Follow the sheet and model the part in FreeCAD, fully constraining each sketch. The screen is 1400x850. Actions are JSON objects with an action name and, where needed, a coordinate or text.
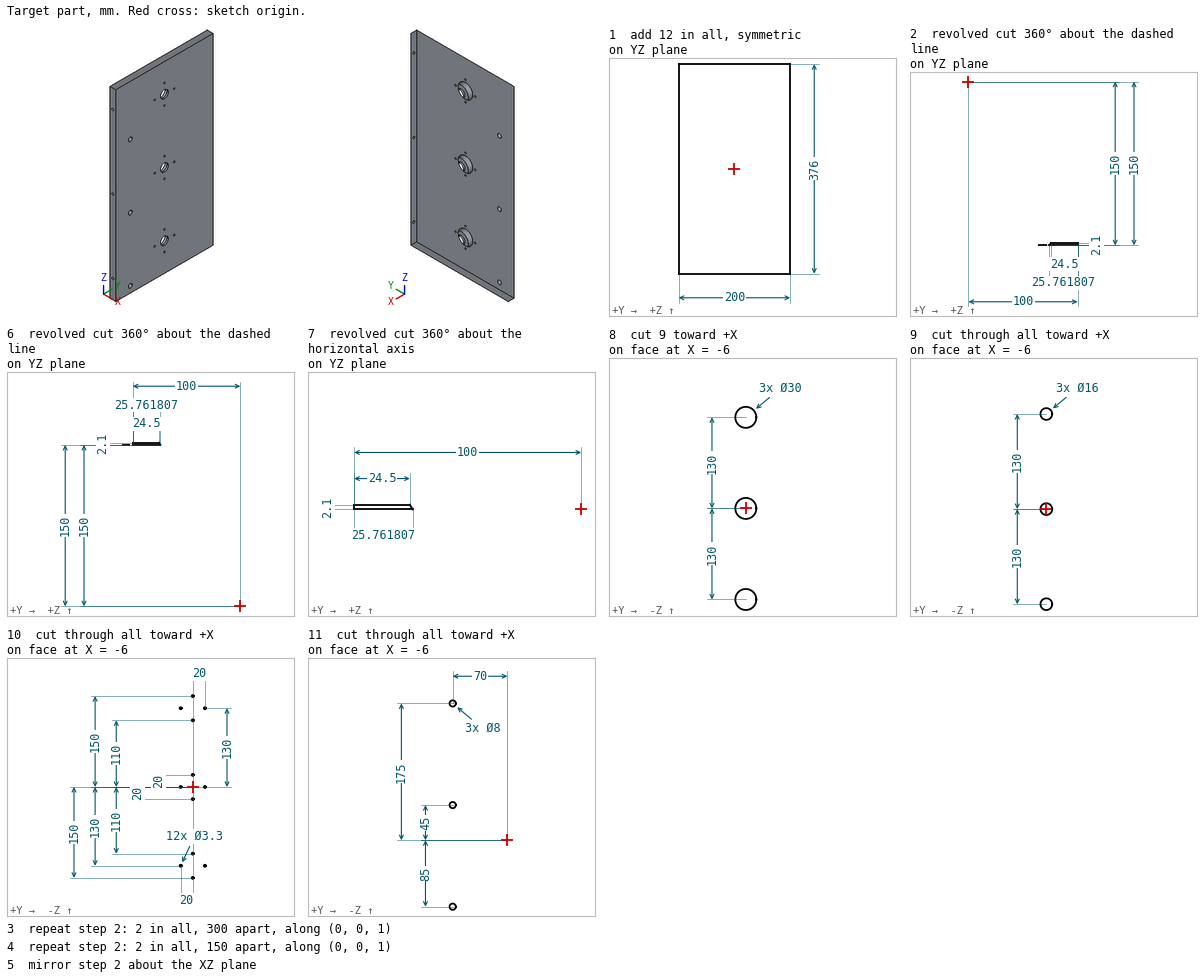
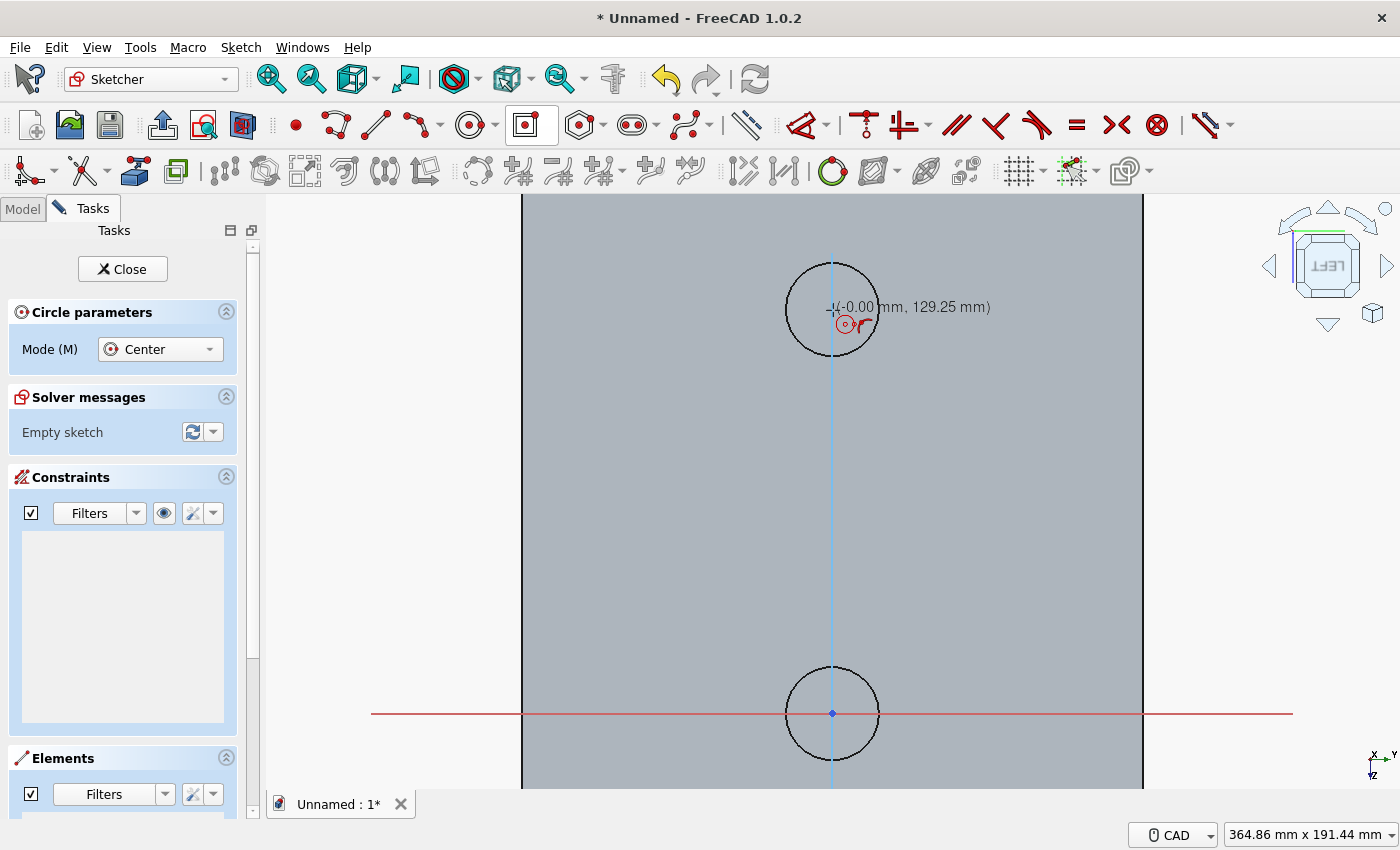
{"action": "left_click", "coordinate": [832, 310]}
{"action": "mouse_move", "coordinate": [850, 292]}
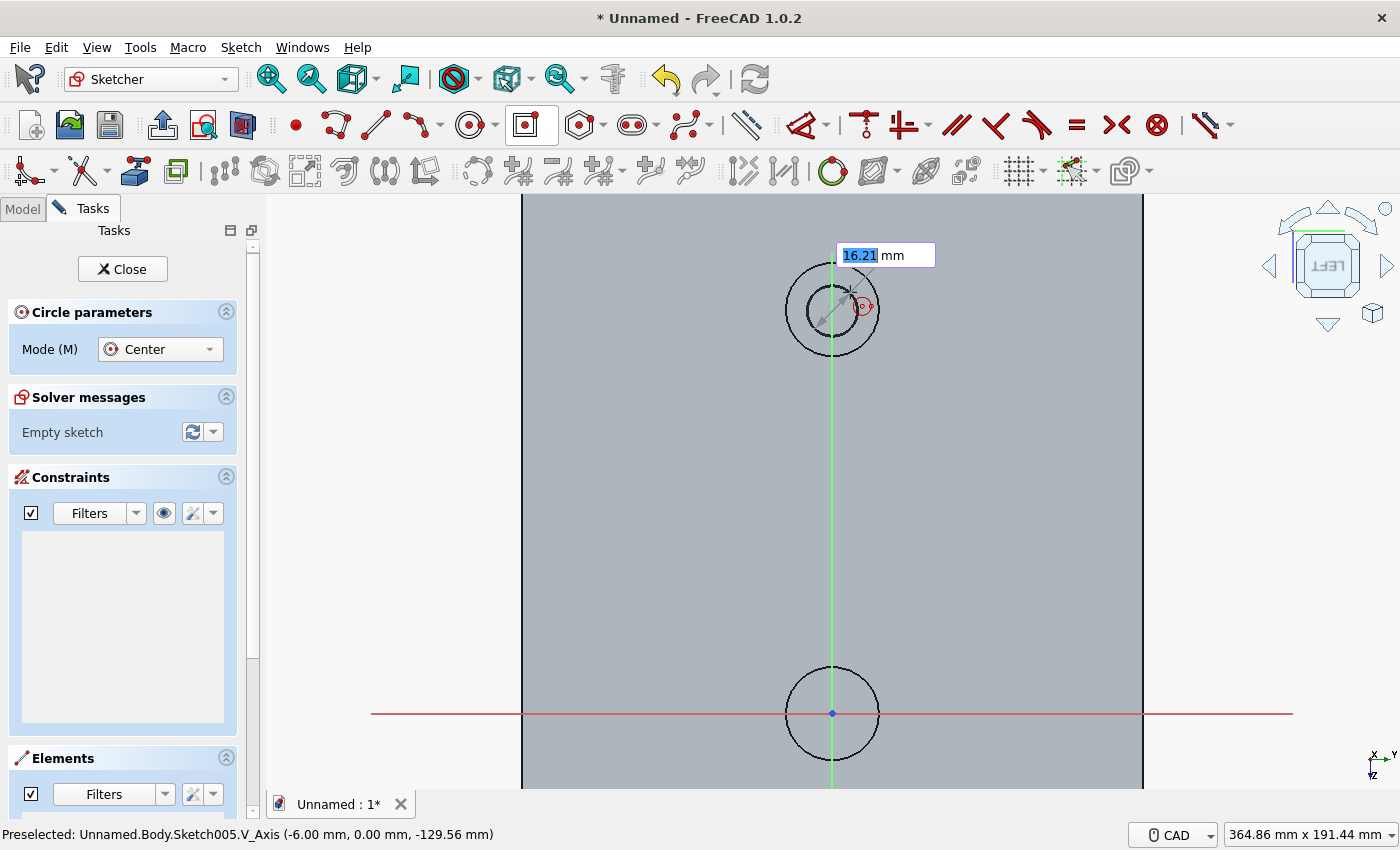
{"action": "type", "text": "16"}
{"action": "key", "text": "Return"}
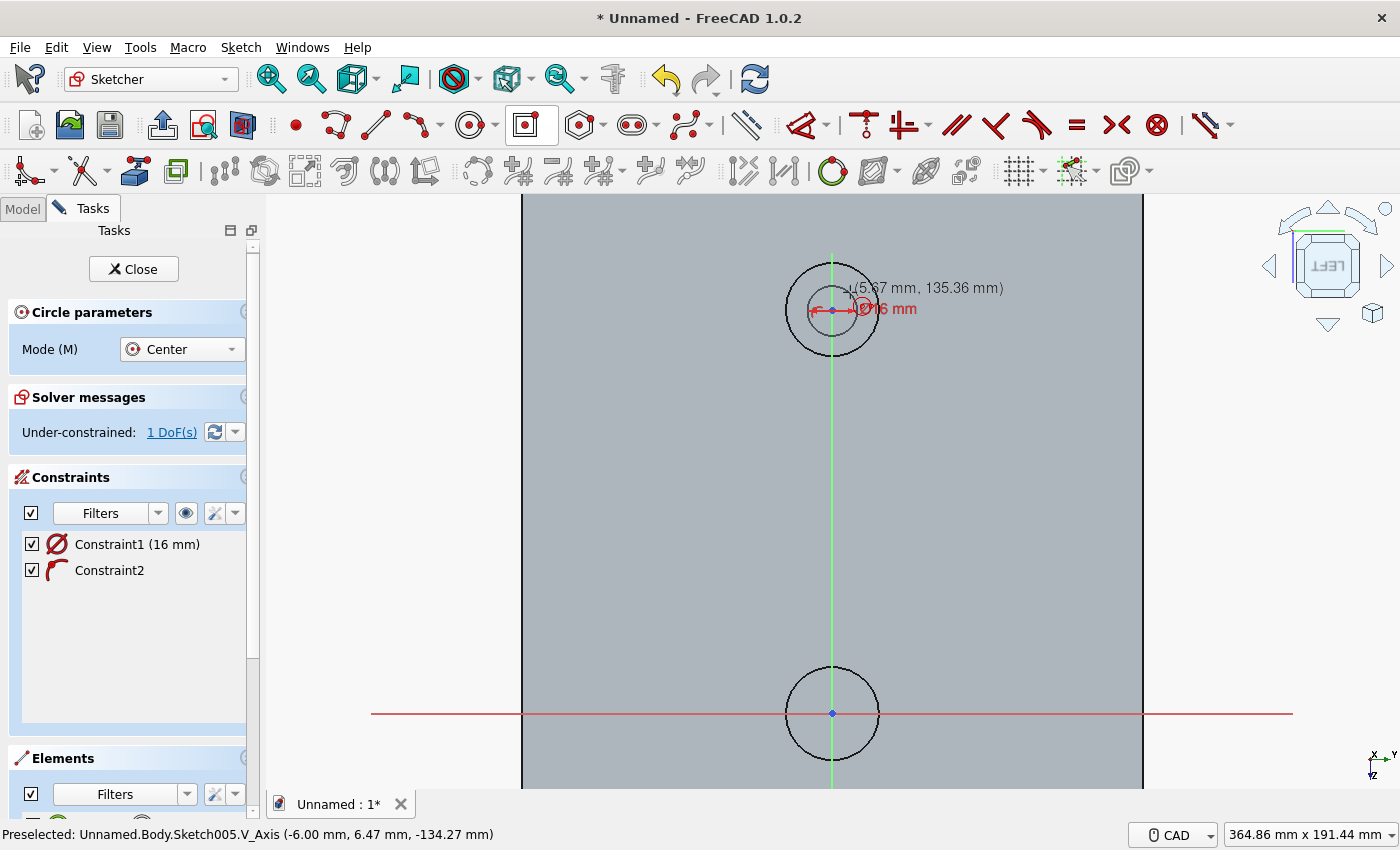
{"action": "left_click", "coordinate": [832, 714]}
{"action": "mouse_move", "coordinate": [850, 696]}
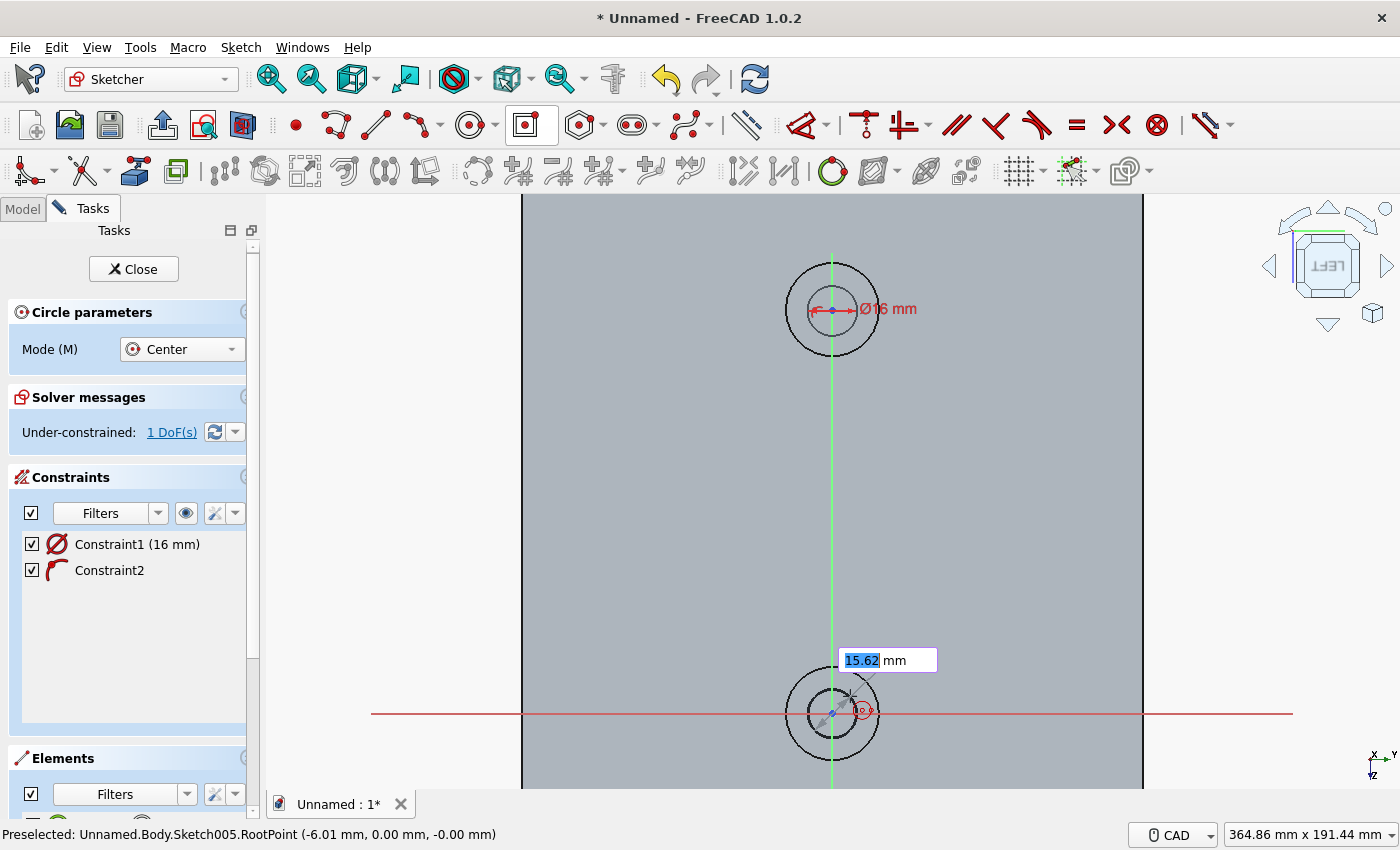
{"action": "type", "text": "16"}
{"action": "key", "text": "Return"}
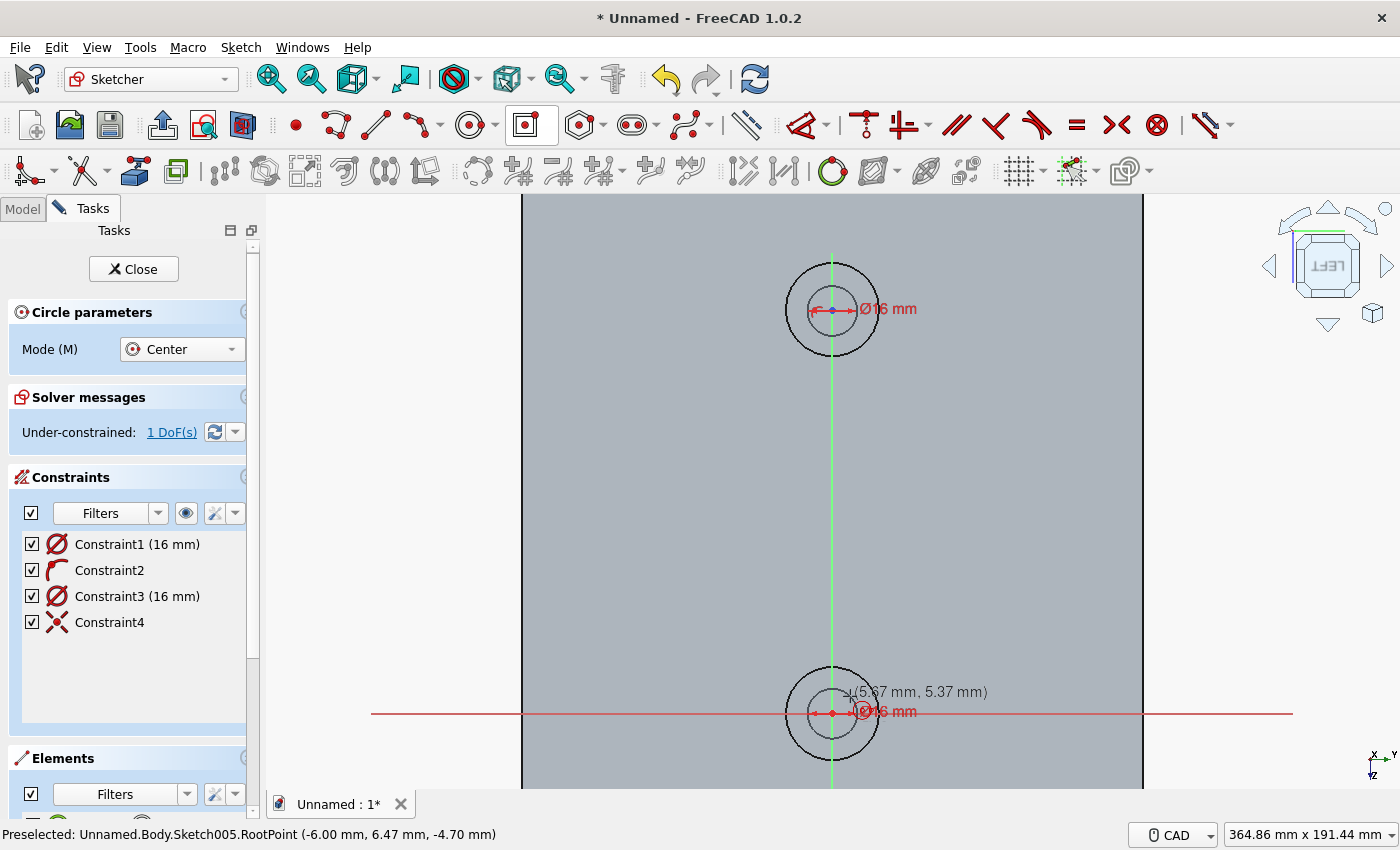
{"action": "scroll", "coordinate": [709, 310], "scroll_direction": "down", "scroll_amount": 4}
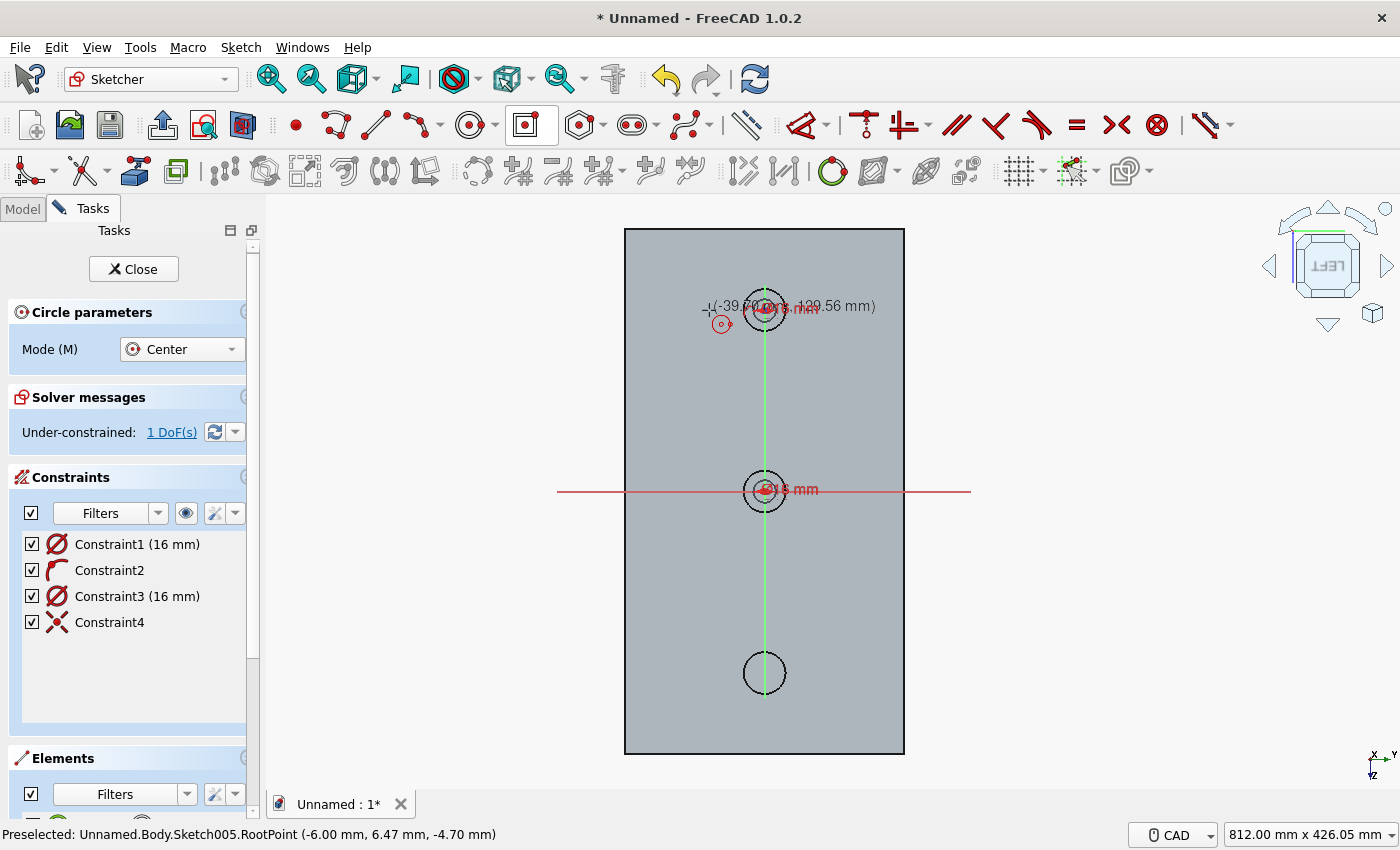
{"action": "scroll", "coordinate": [765, 673], "scroll_direction": "up", "scroll_amount": 4}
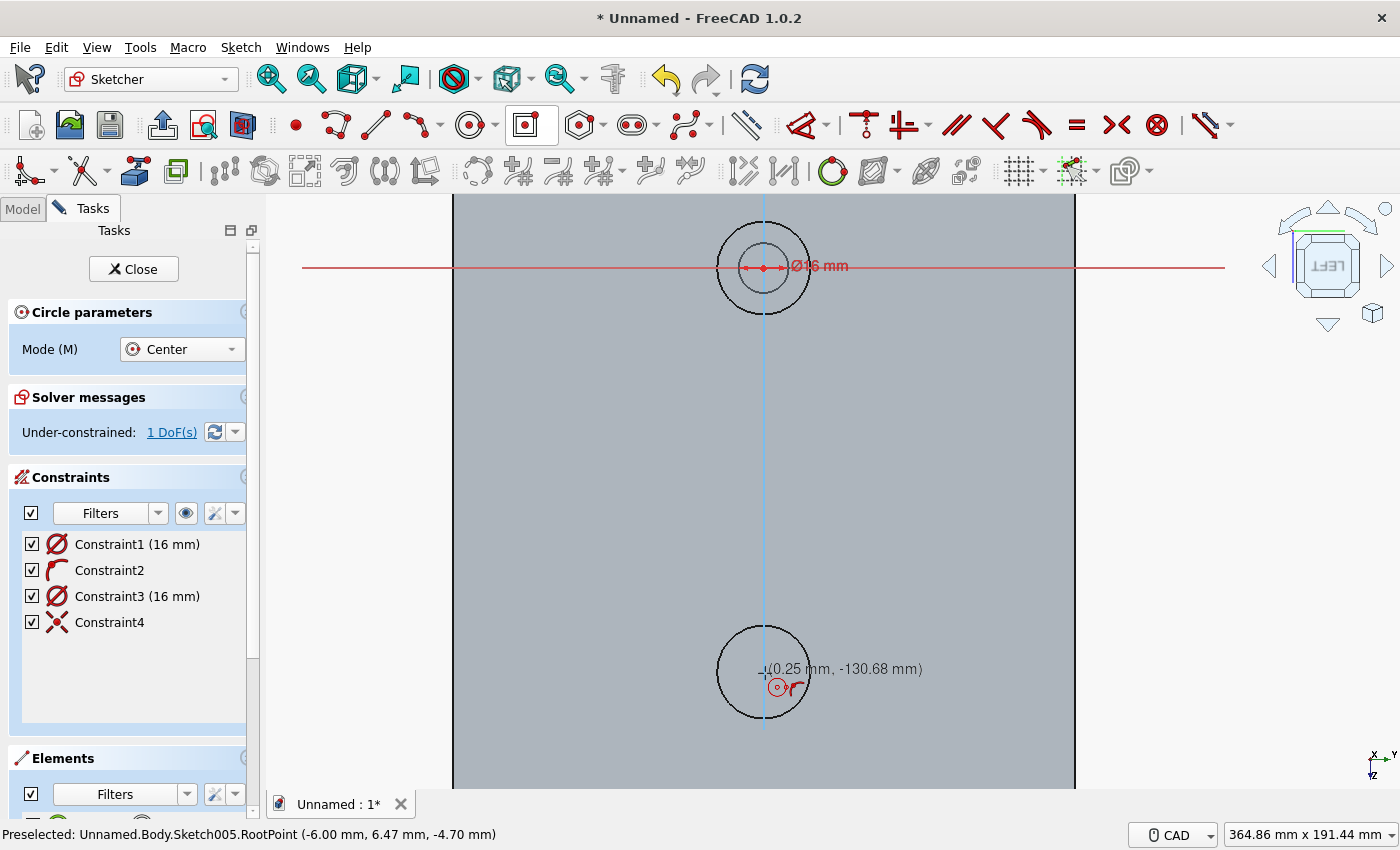
{"action": "left_click", "coordinate": [764, 672]}
{"action": "mouse_move", "coordinate": [781, 655]}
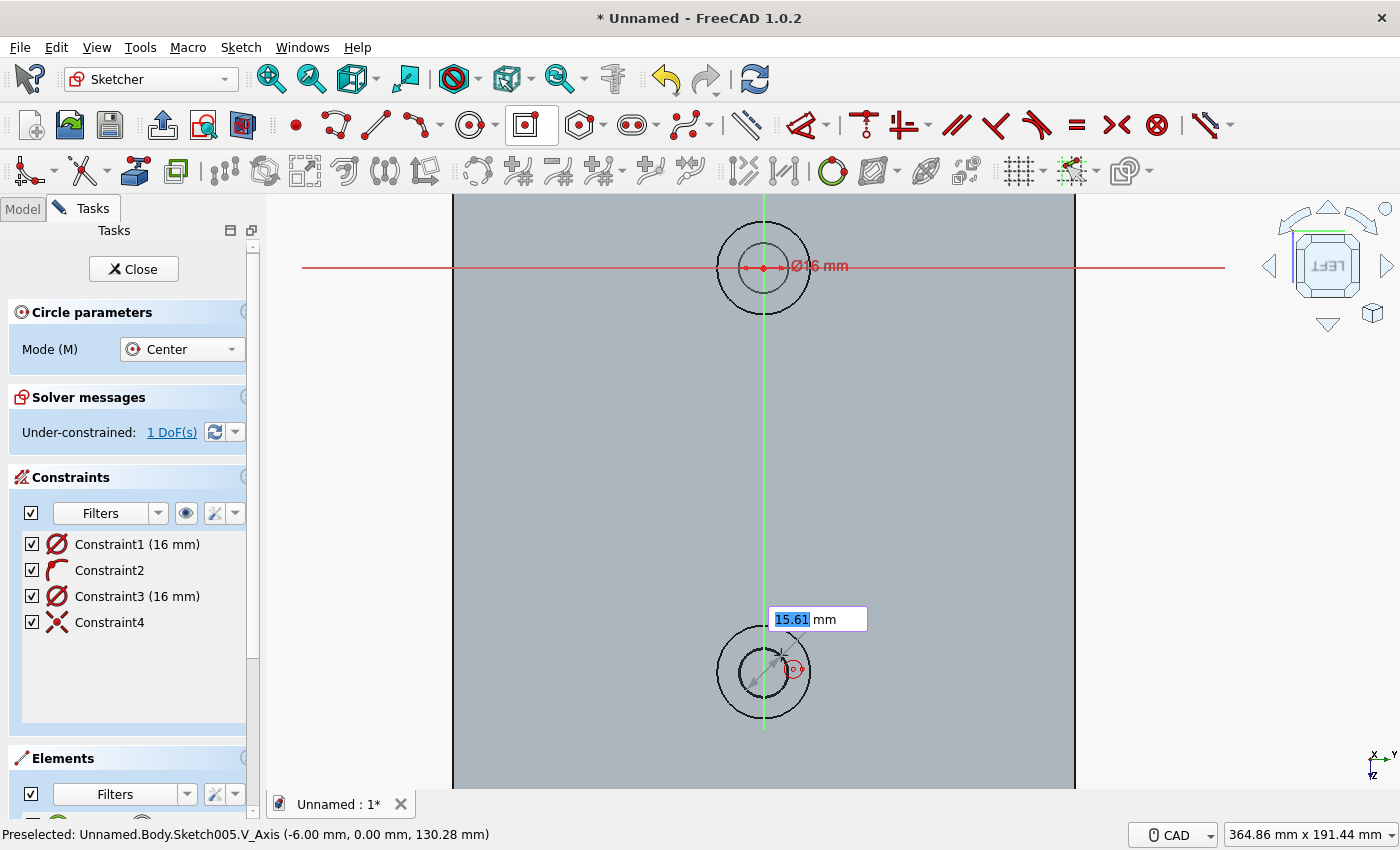
{"action": "type", "text": "16"}
{"action": "key", "text": "Return"}
{"action": "key", "text": "Escape"}